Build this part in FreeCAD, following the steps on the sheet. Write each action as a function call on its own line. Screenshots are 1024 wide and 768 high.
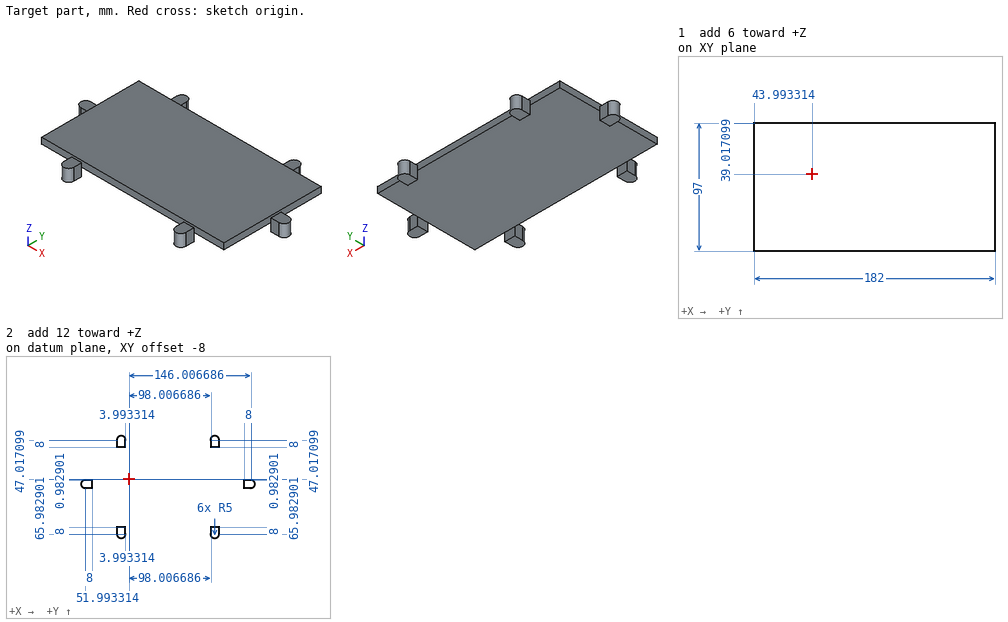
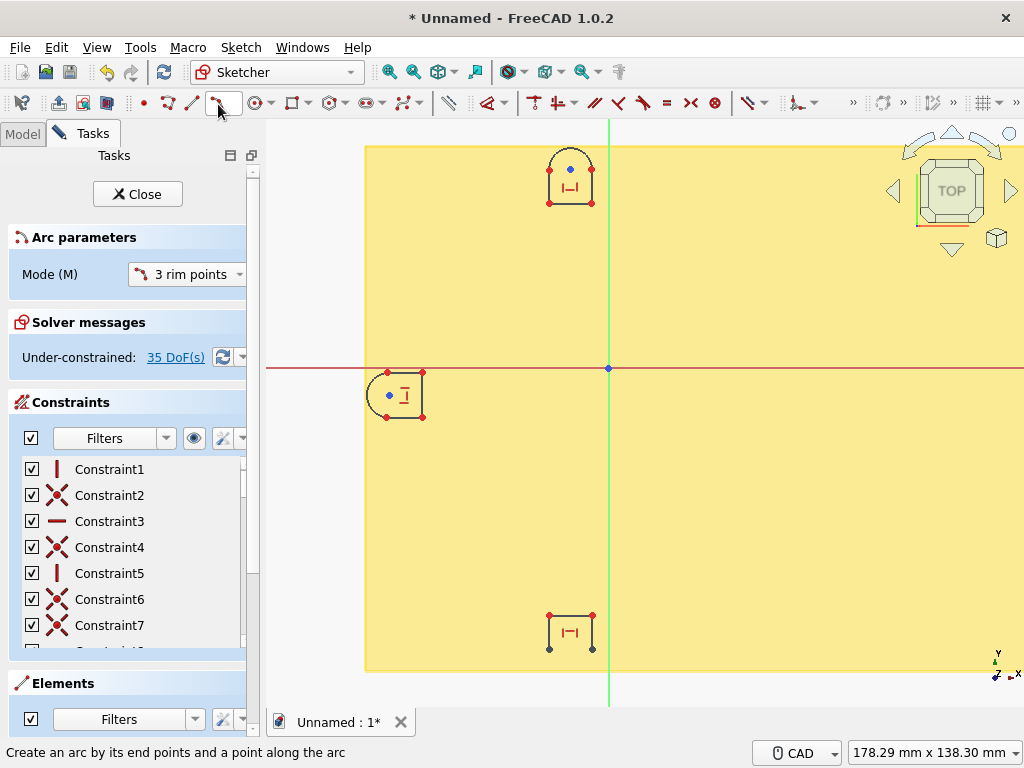
click(549, 650)
click(592, 650)
click(571, 670)
key(Escape)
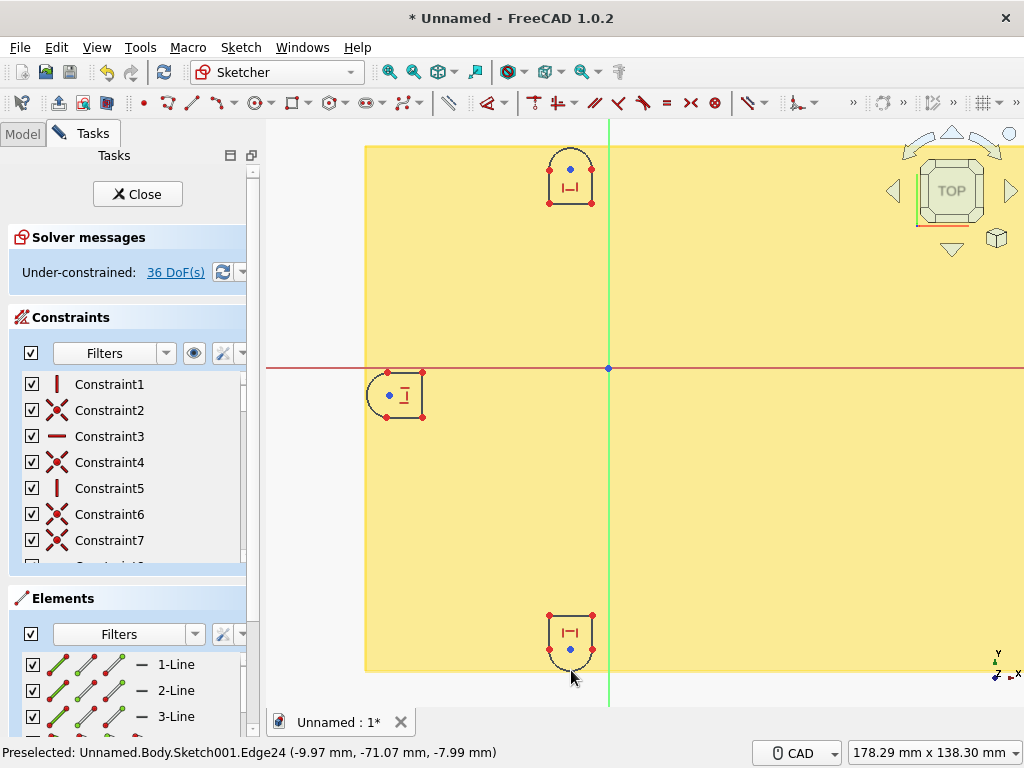
scroll(387, 416, down, 4)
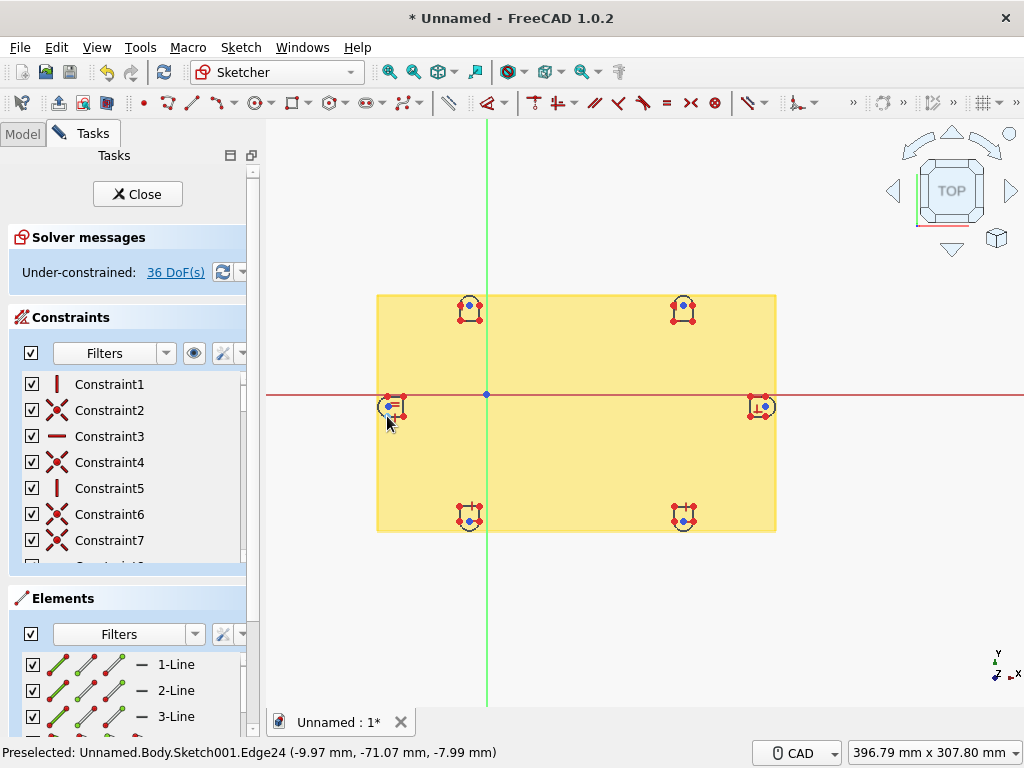
scroll(693, 517, up, 6)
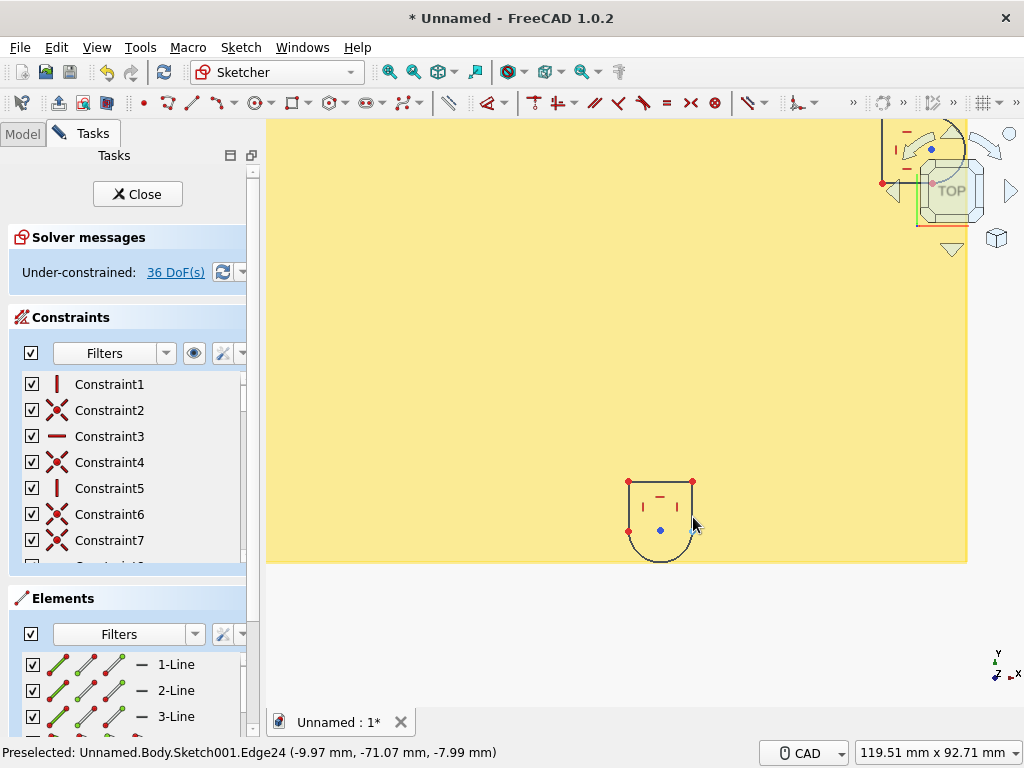
click(692, 517)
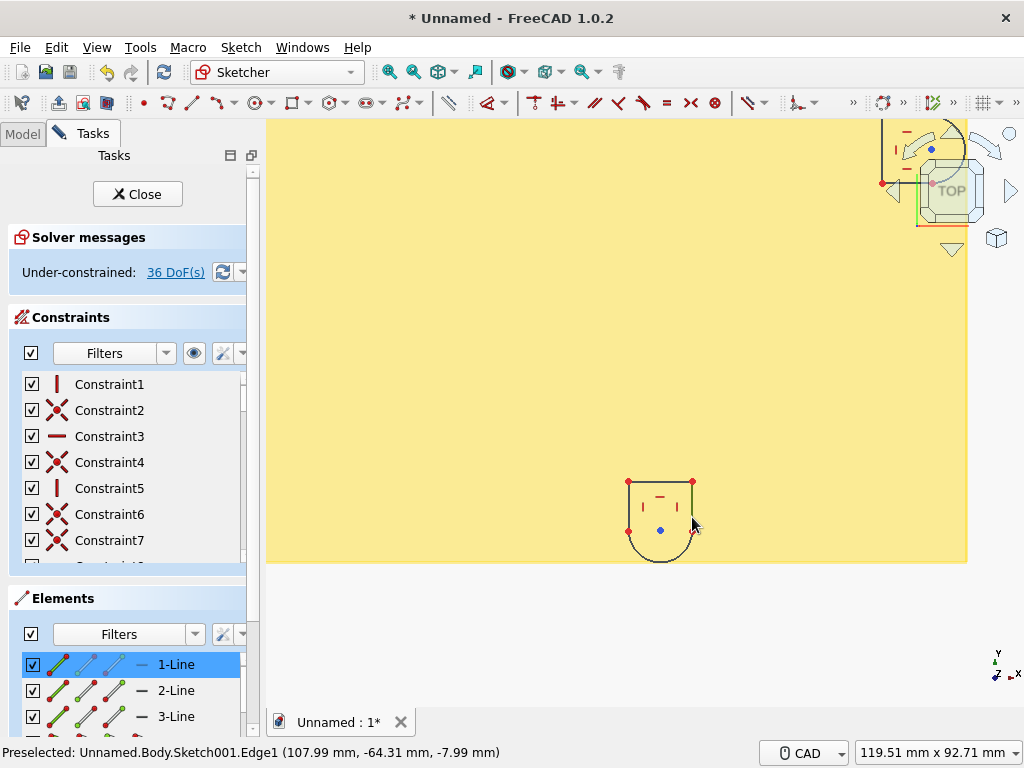
click(642, 557)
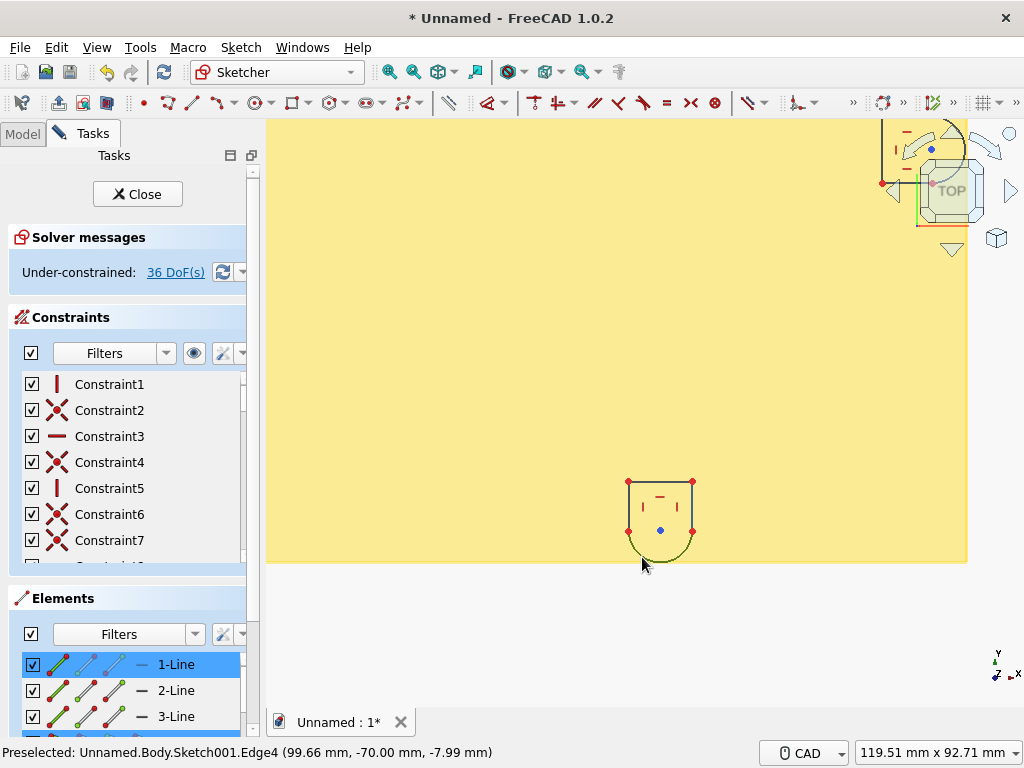
click(644, 104)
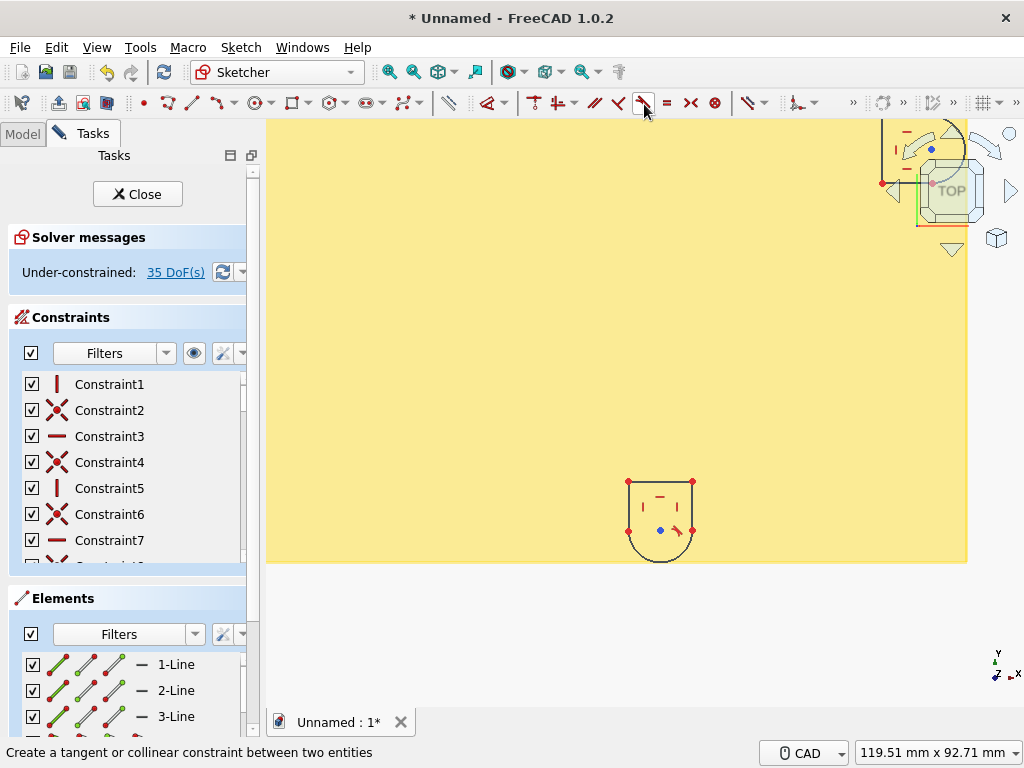
click(629, 497)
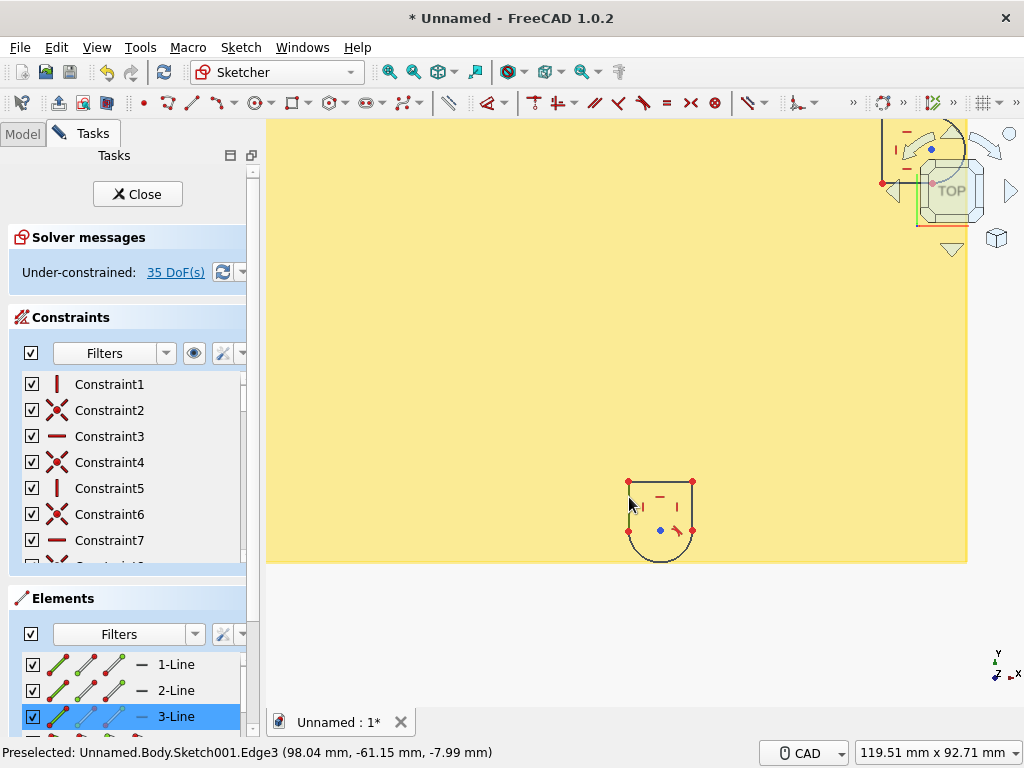
click(642, 557)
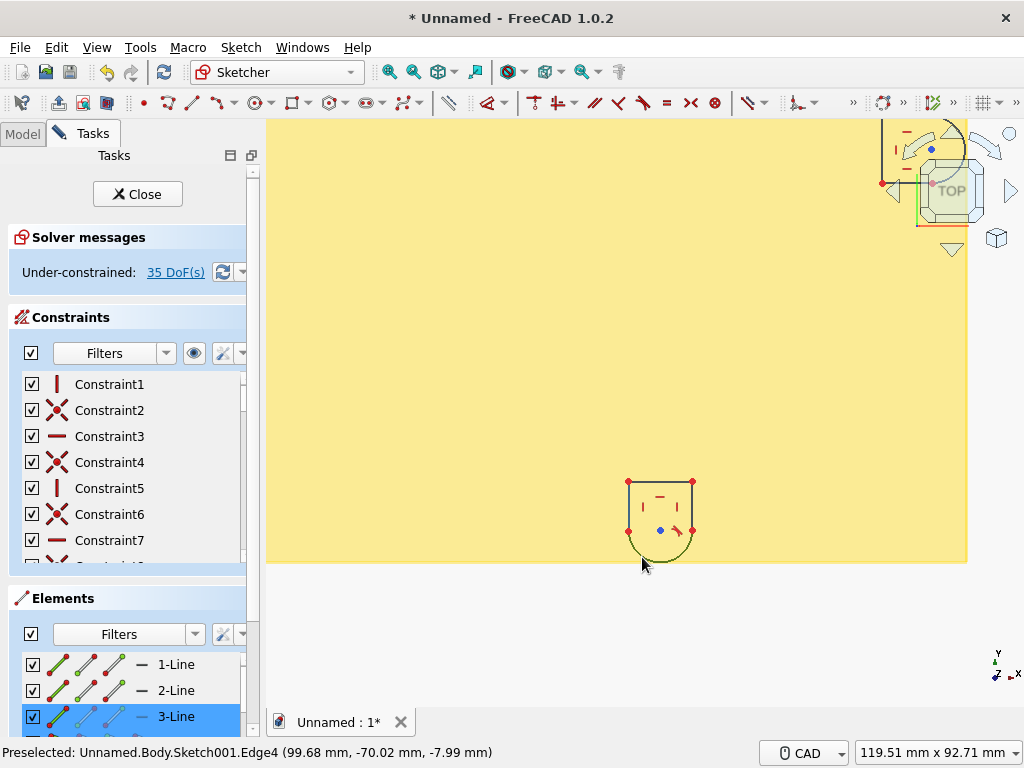
click(644, 104)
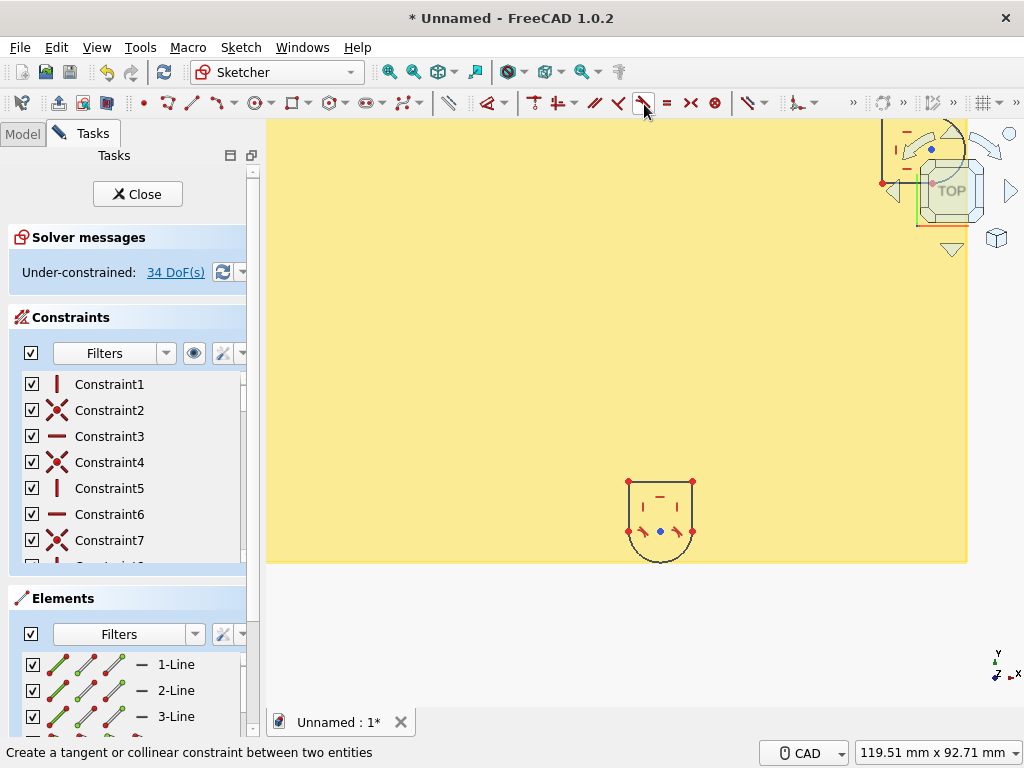
scroll(693, 518, down, 6)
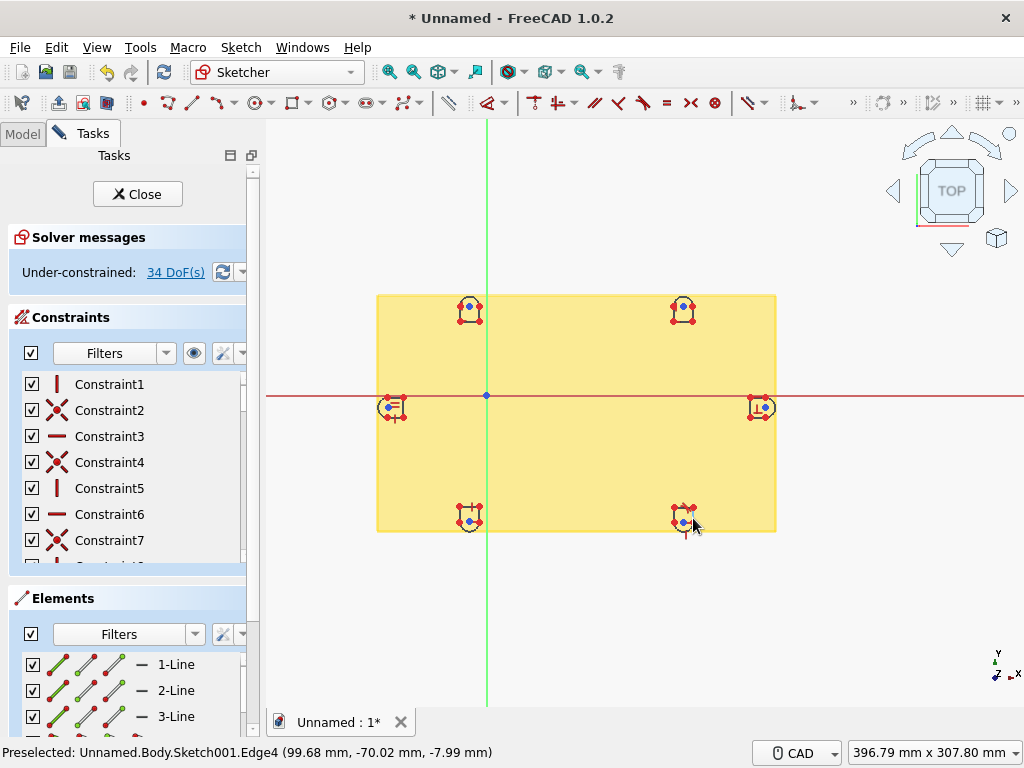
scroll(761, 398, up, 10)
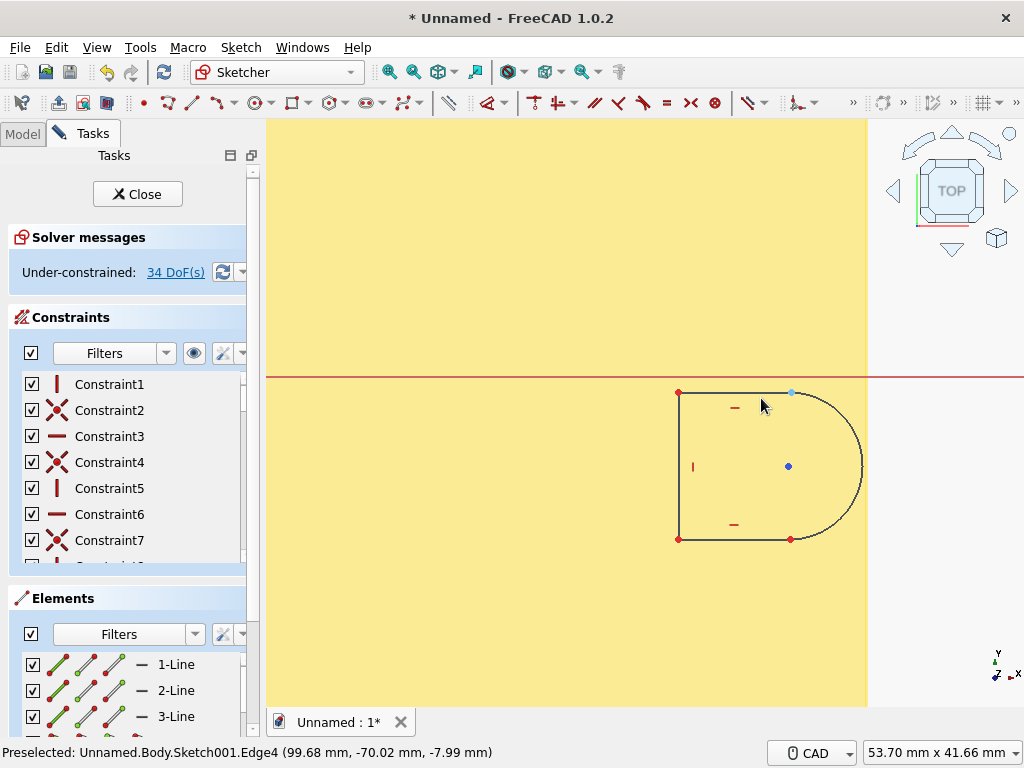
click(758, 393)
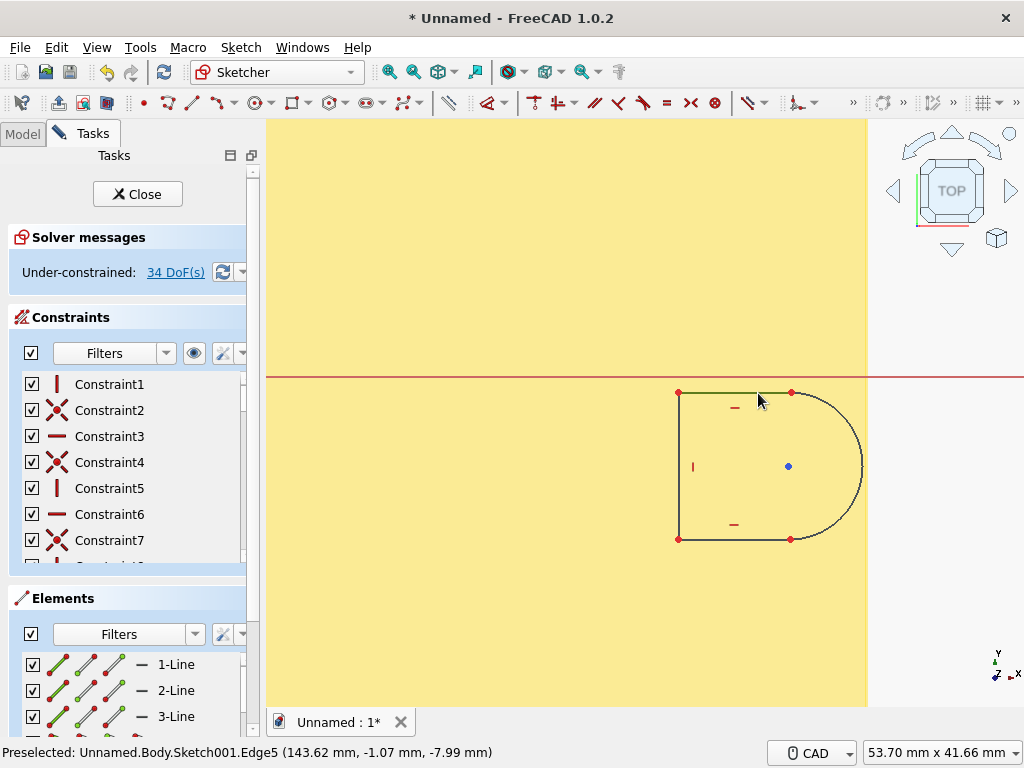
scroll(762, 398, down, 10)